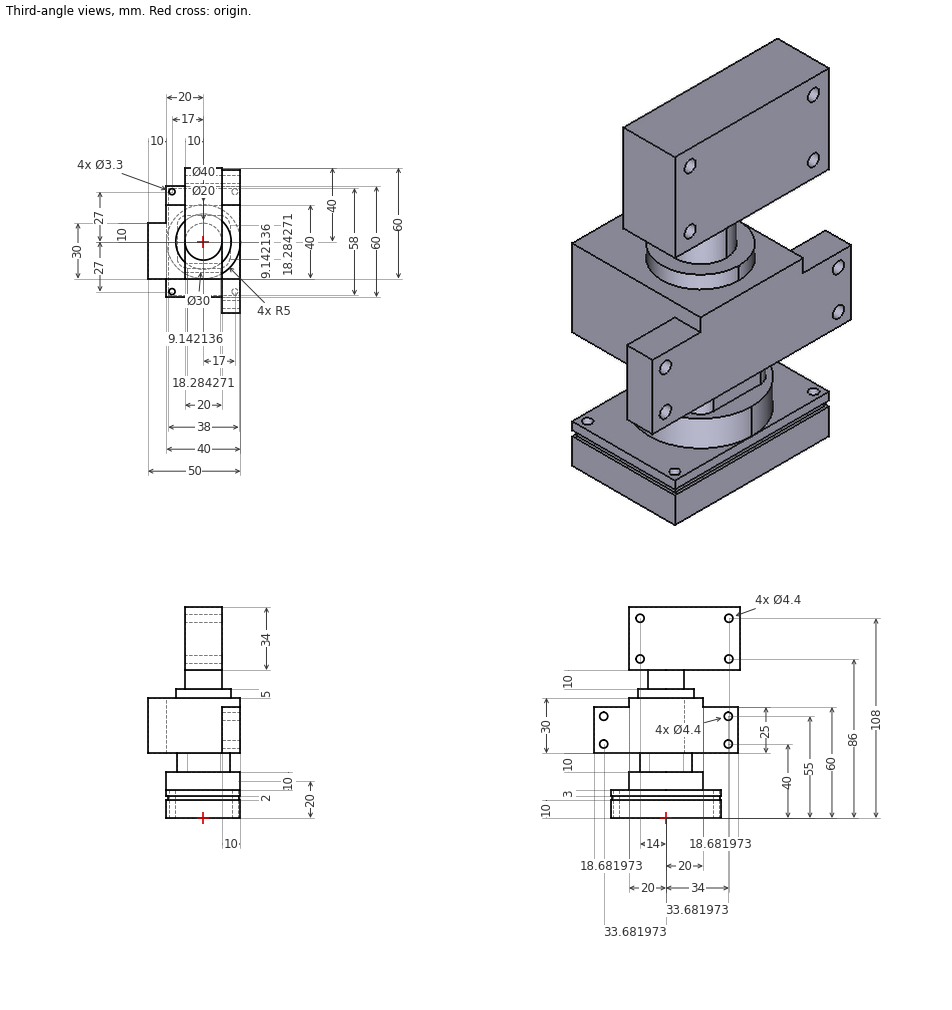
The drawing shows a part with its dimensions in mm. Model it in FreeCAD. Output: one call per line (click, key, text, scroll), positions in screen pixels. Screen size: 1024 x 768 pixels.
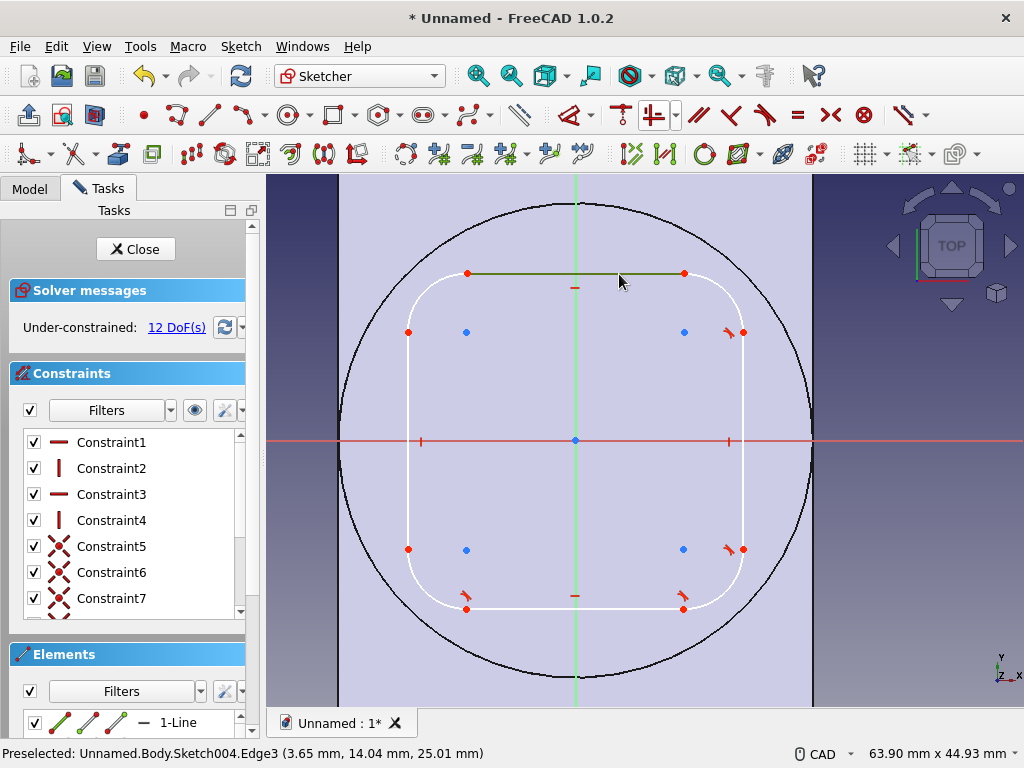
click(737, 306)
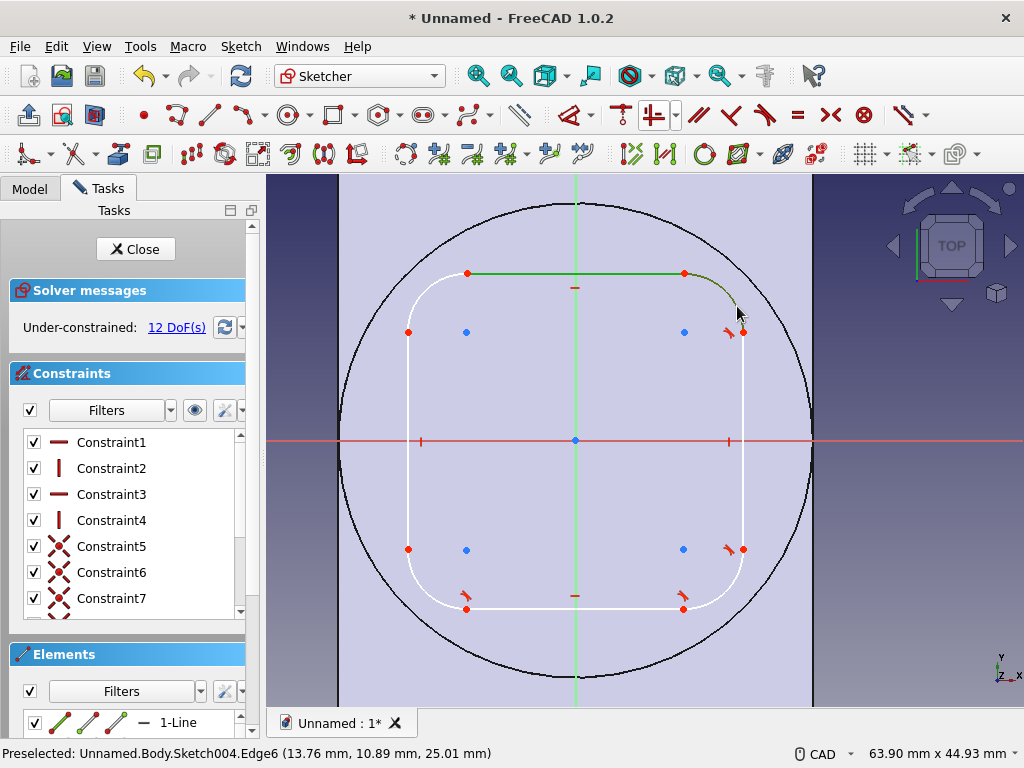
key(t)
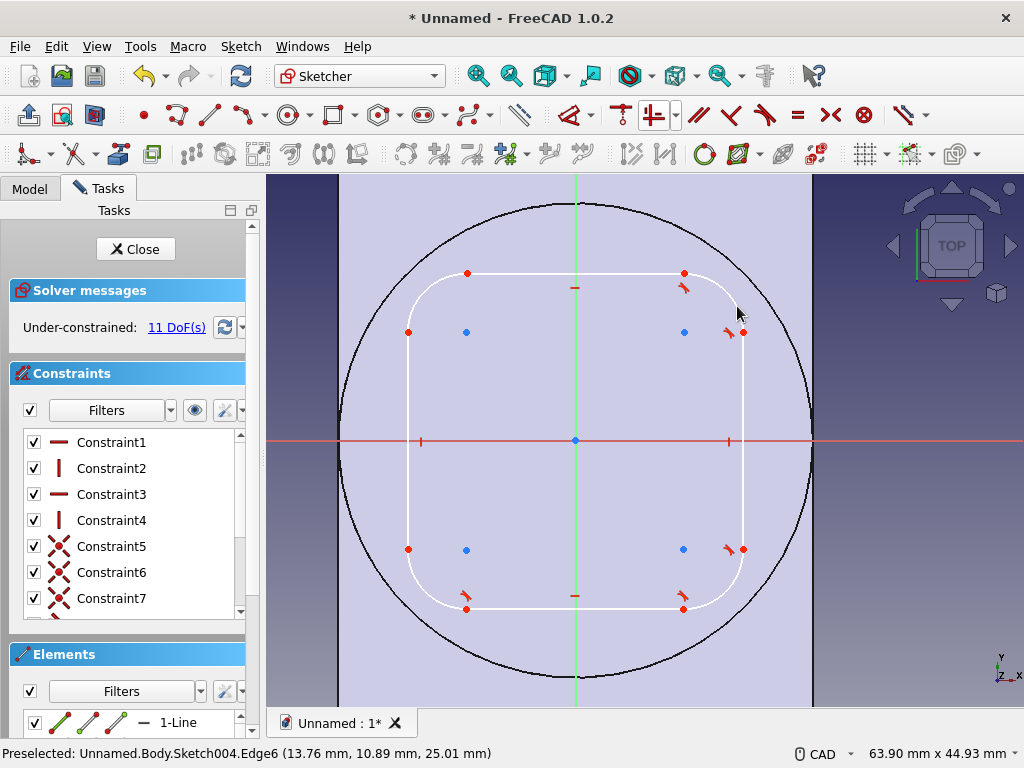
click(619, 274)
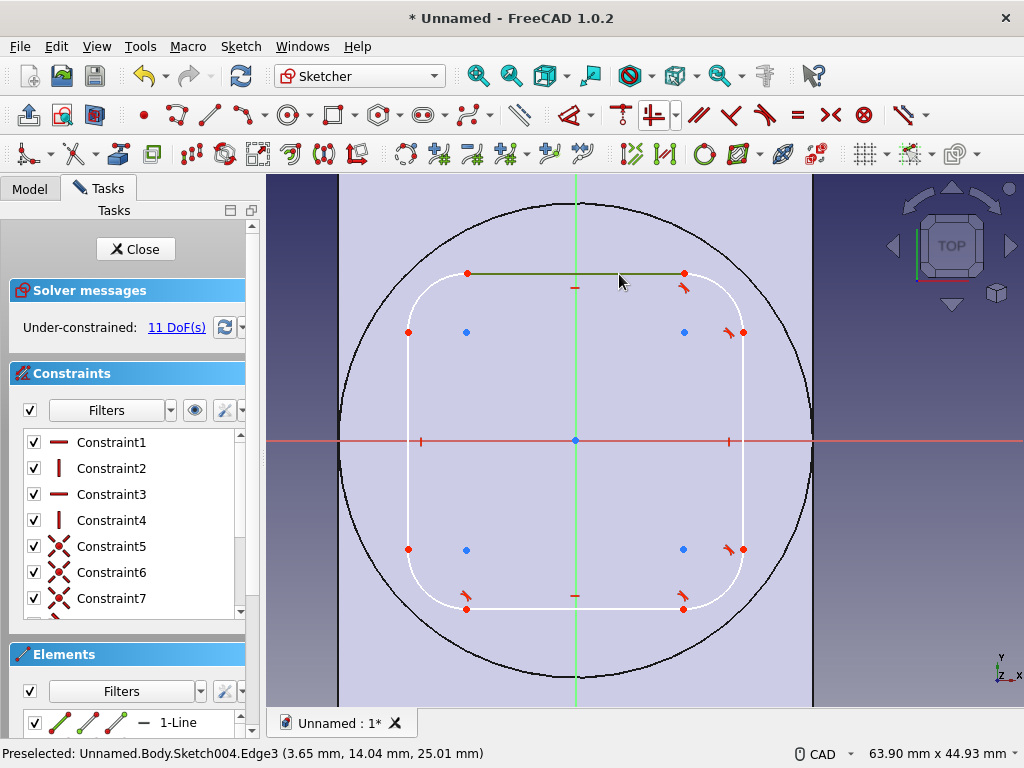
click(440, 280)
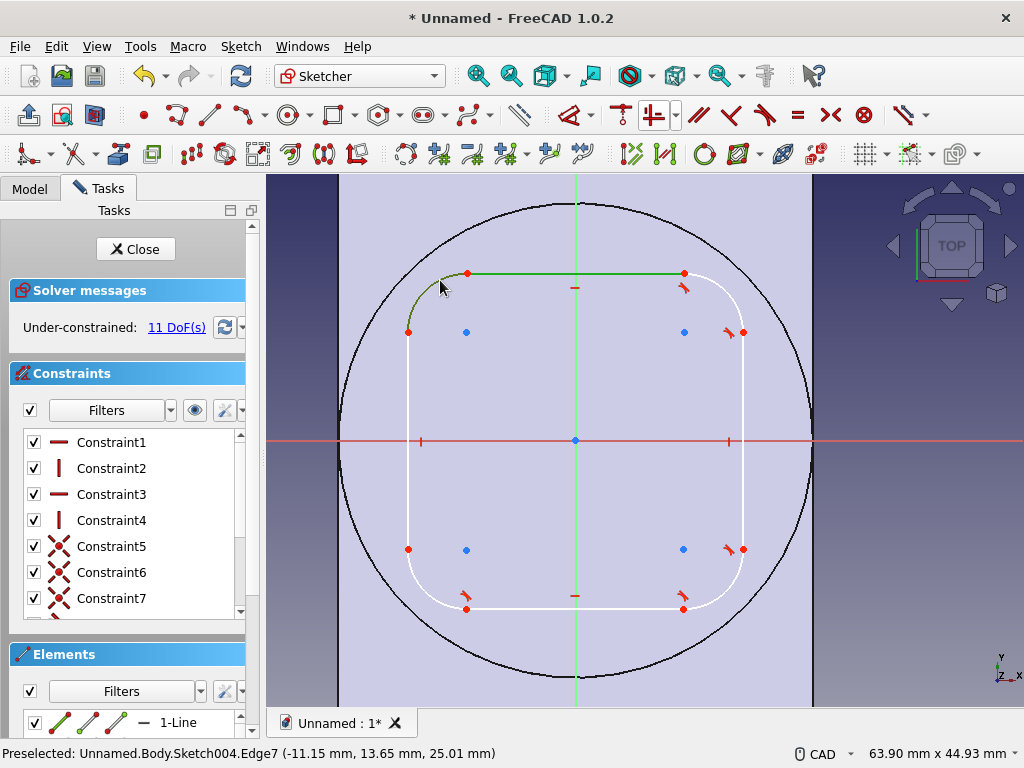
key(t)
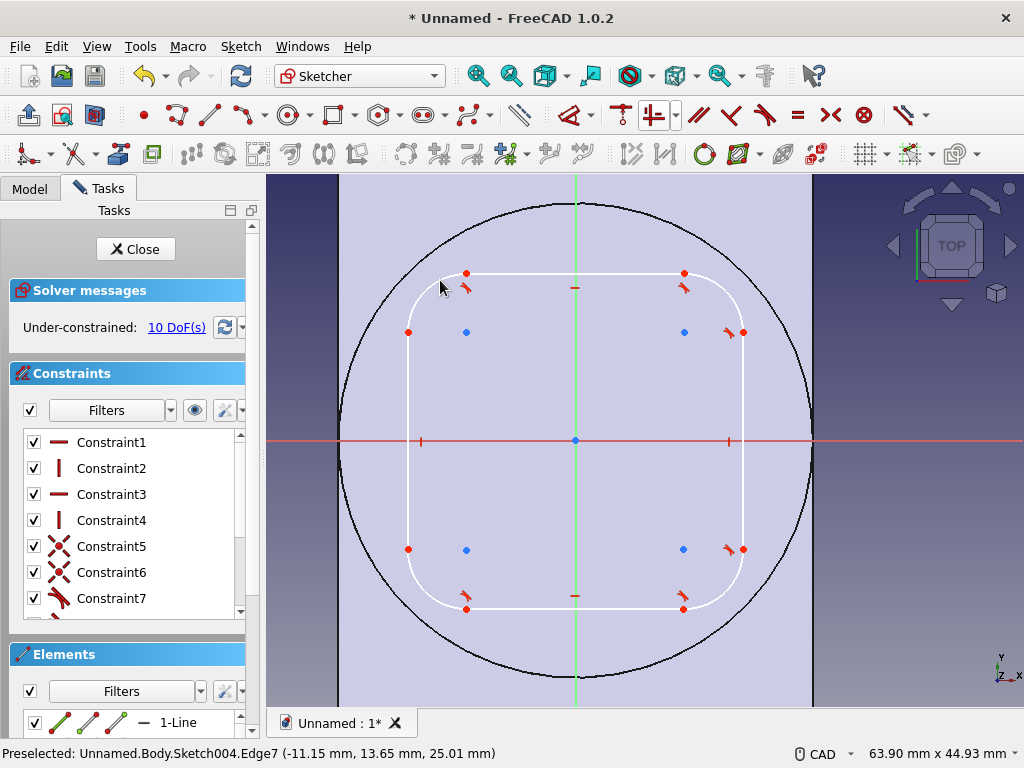
click(408, 398)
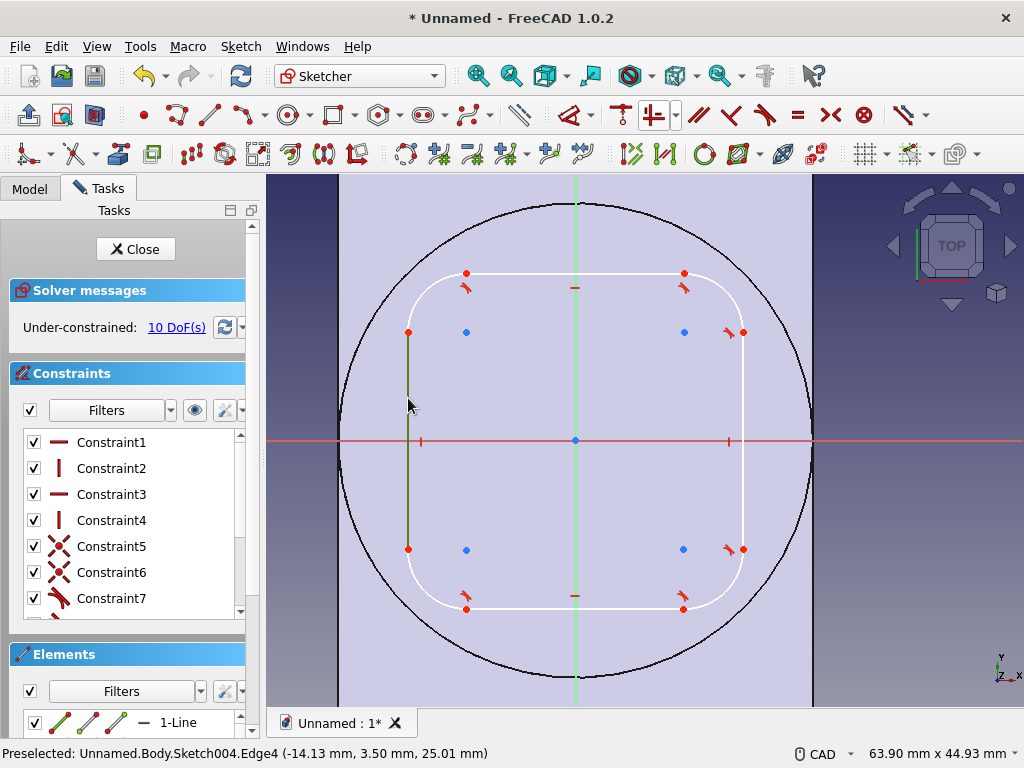
click(440, 280)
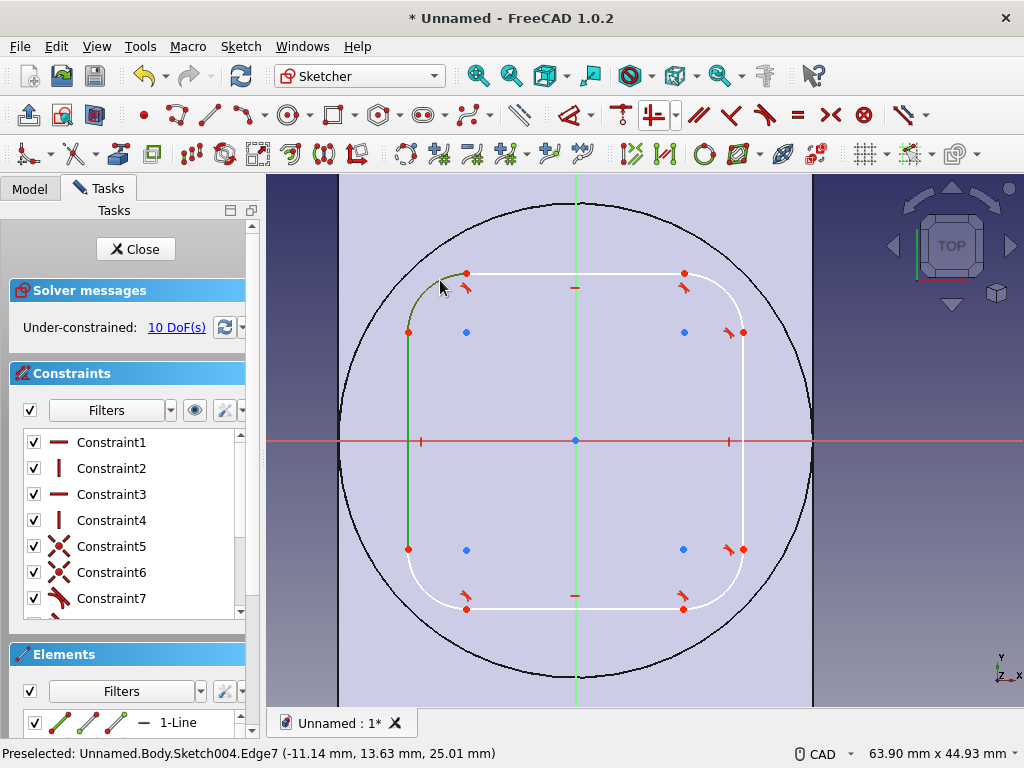
key(t)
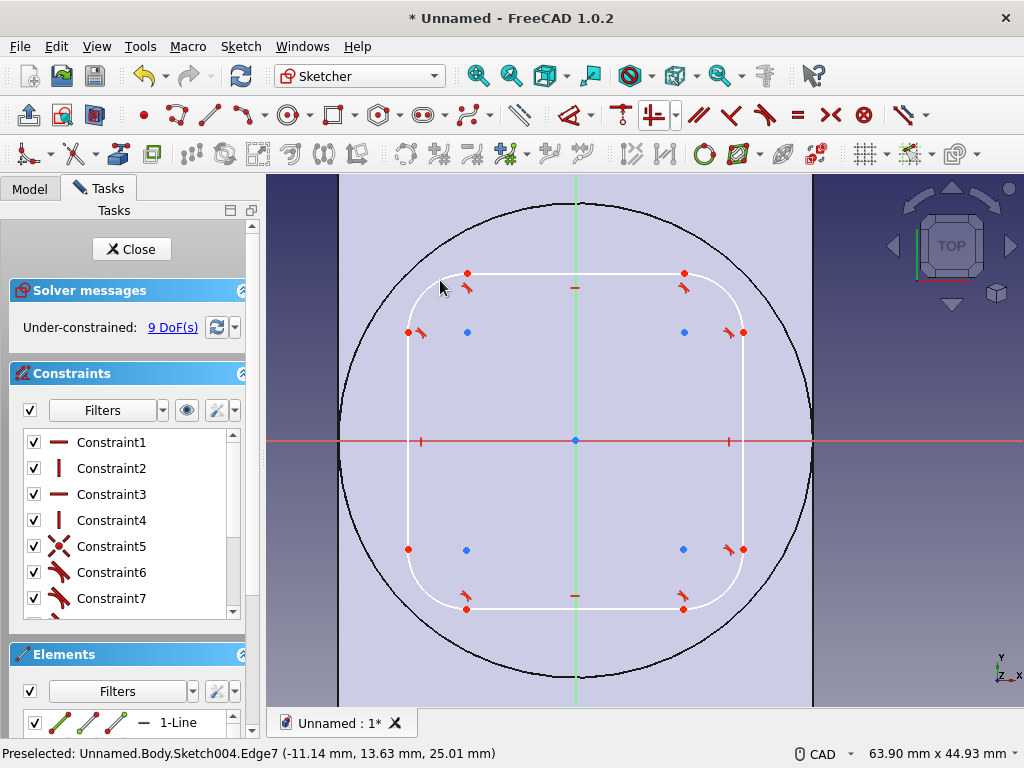
click(408, 398)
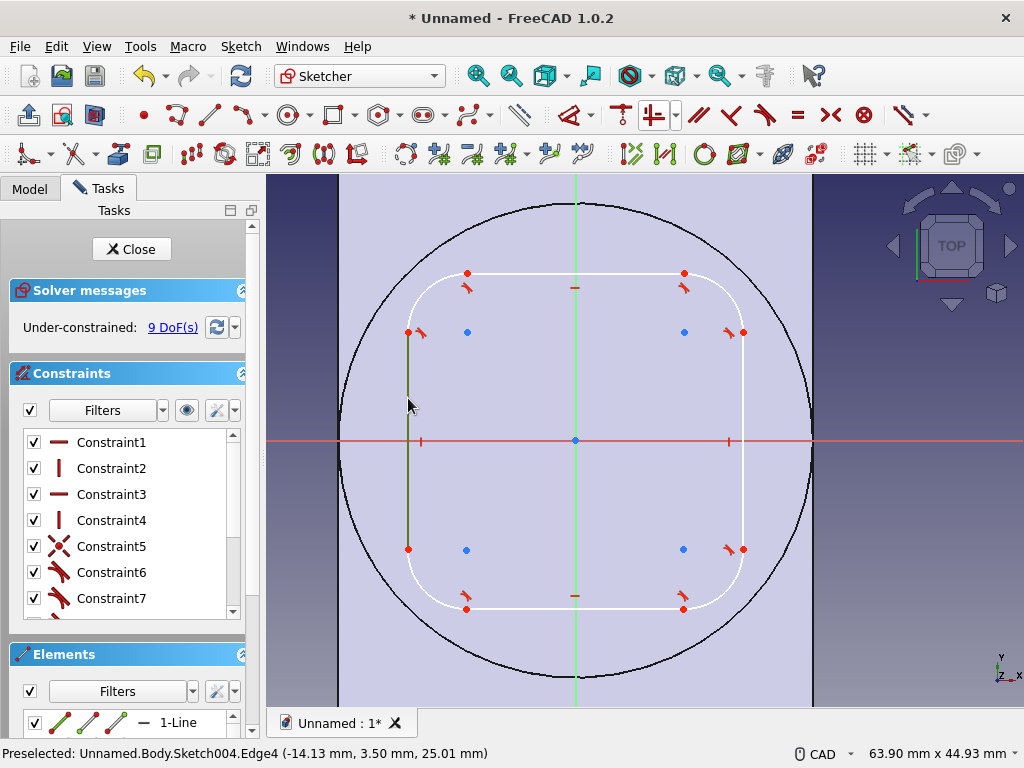
click(414, 577)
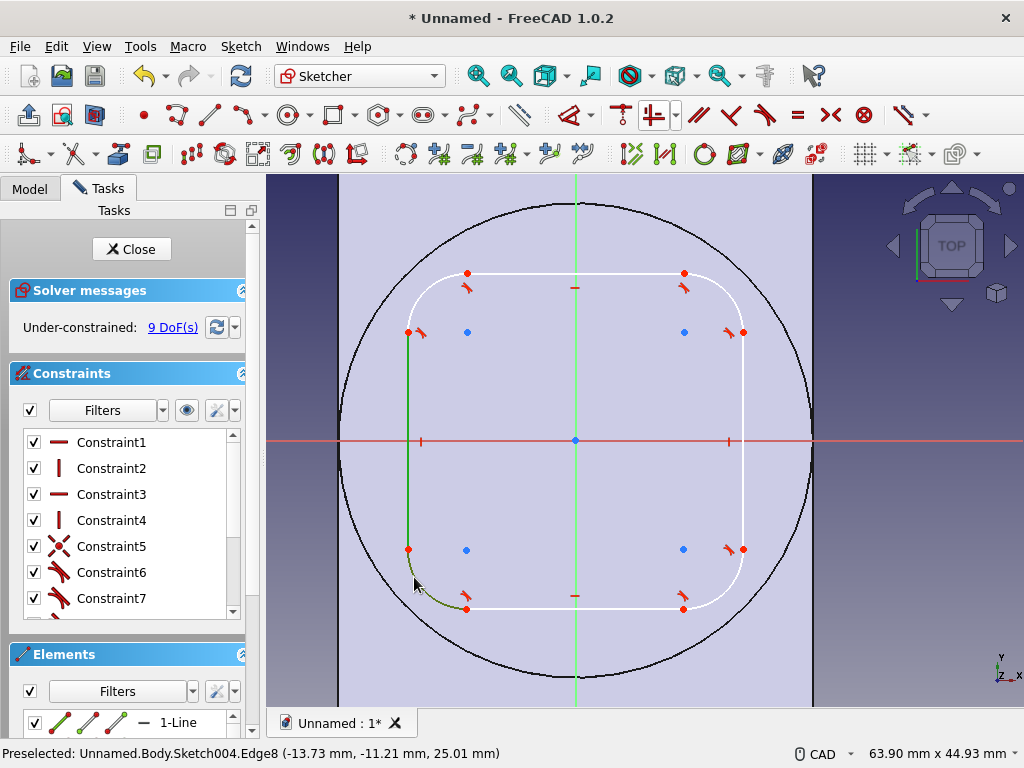
click(765, 116)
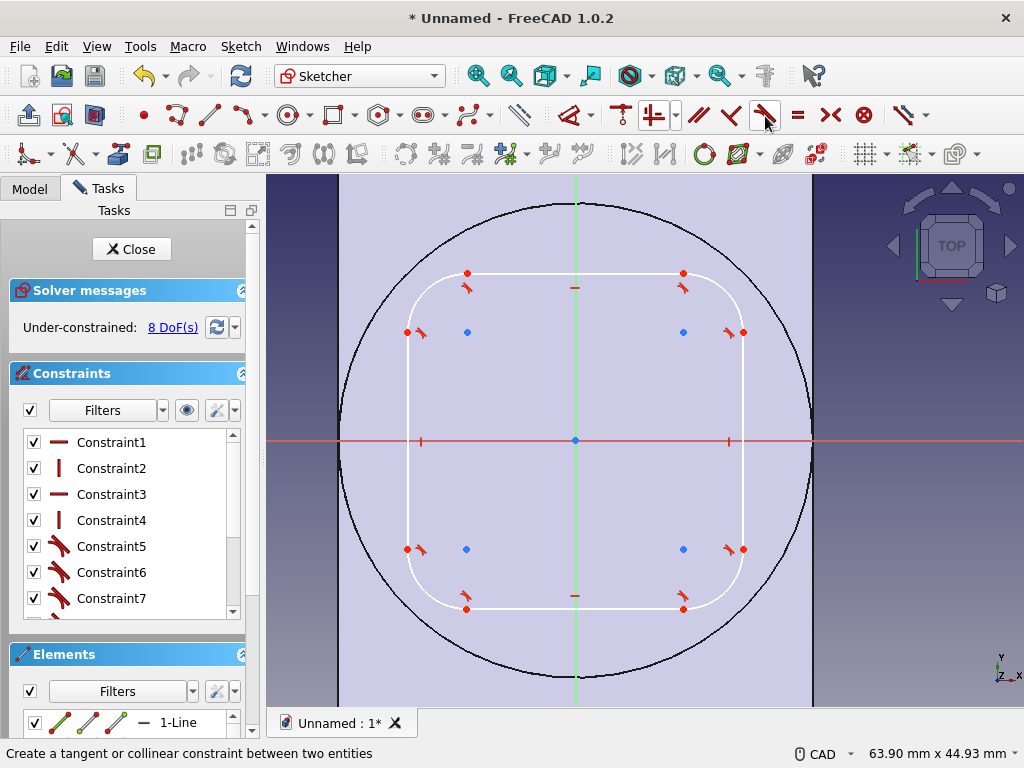
click(711, 603)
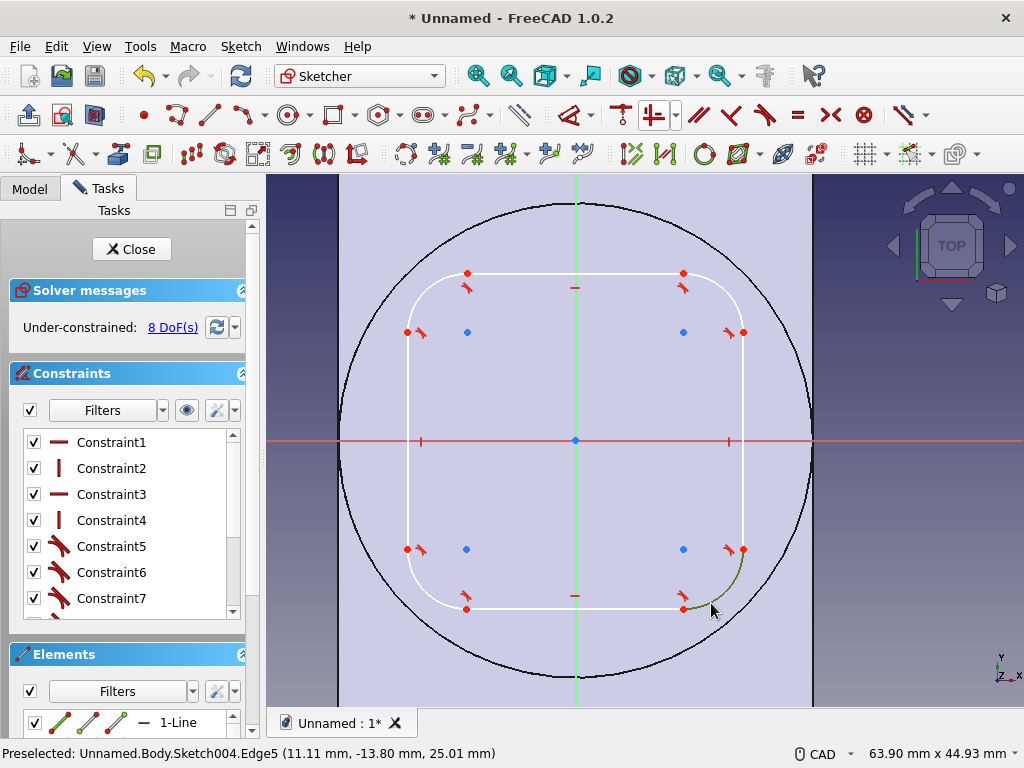
click(737, 306)